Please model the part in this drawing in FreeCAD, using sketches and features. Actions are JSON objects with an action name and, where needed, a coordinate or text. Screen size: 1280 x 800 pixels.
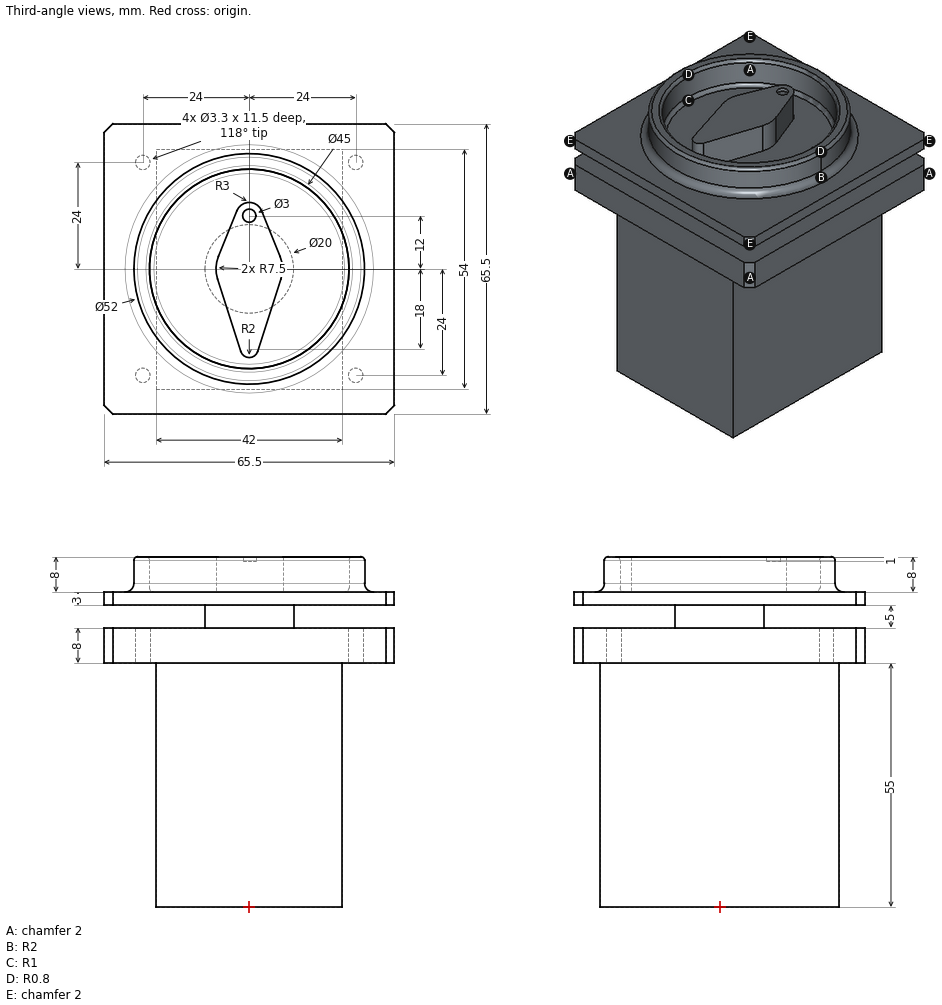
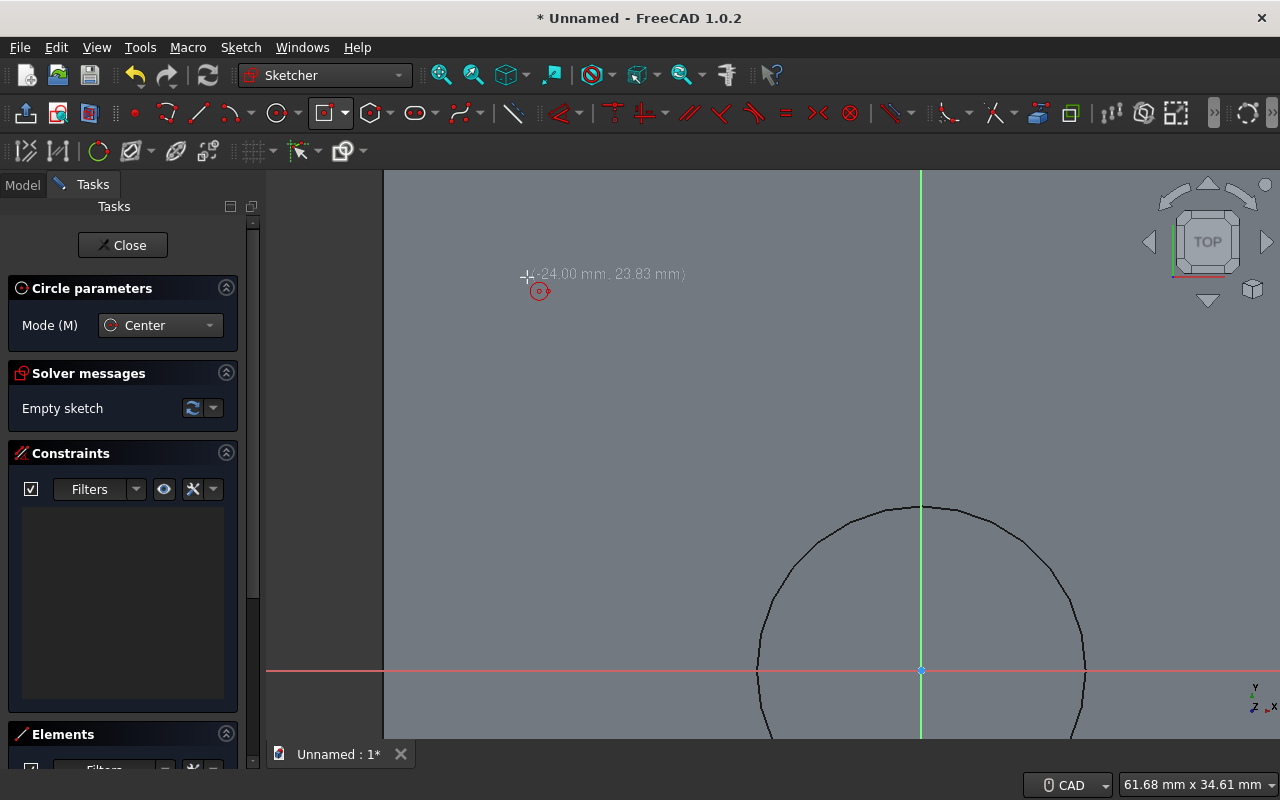
{"action": "left_click", "coordinate": [527, 276]}
{"action": "mouse_move", "coordinate": [546, 257]}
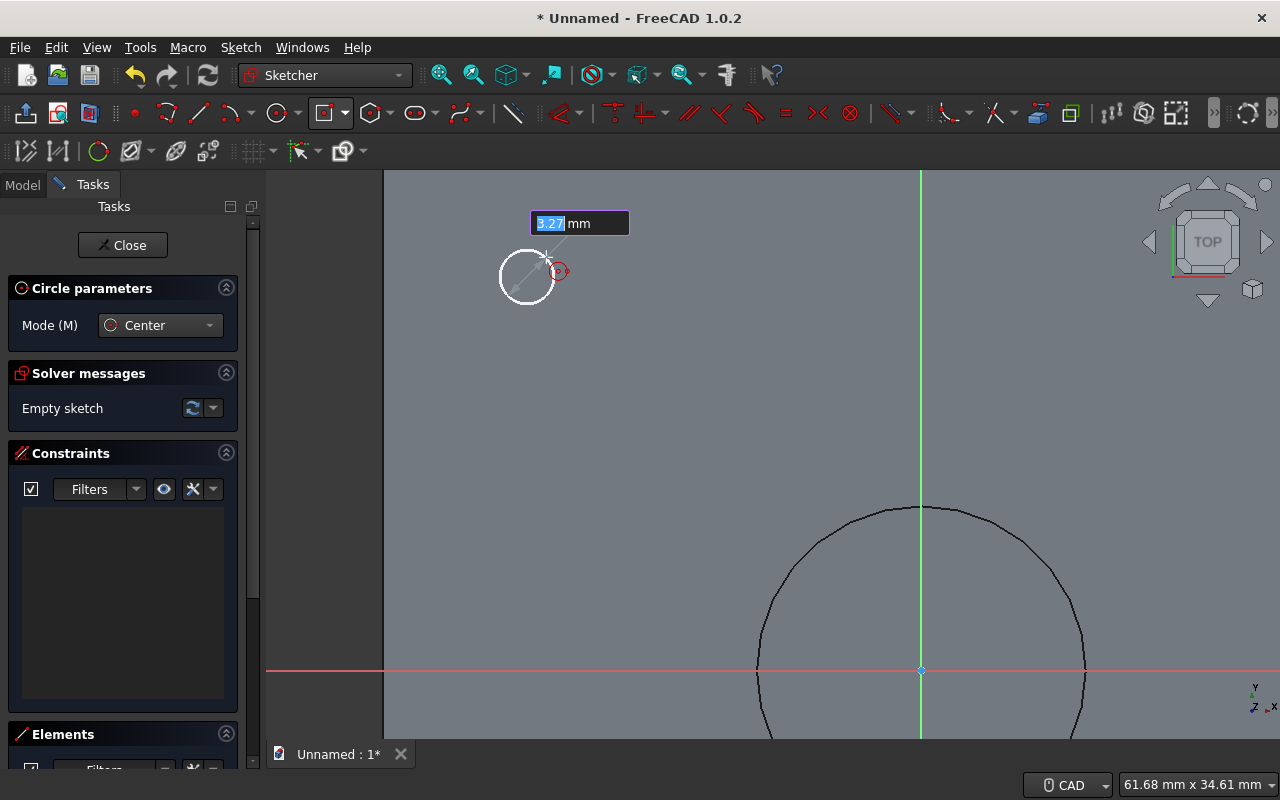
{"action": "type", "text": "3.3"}
{"action": "key", "text": "Return"}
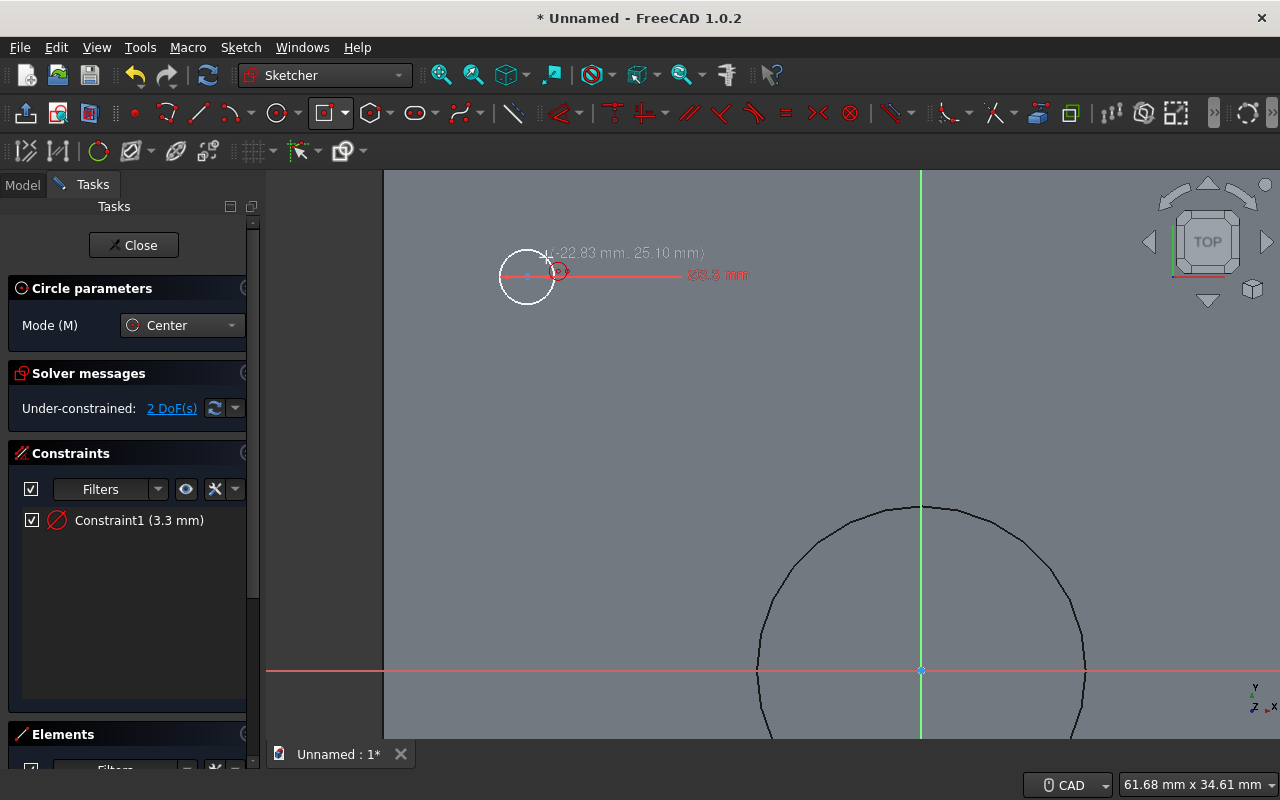
{"action": "scroll", "coordinate": [528, 278], "scroll_direction": "down", "scroll_amount": 4}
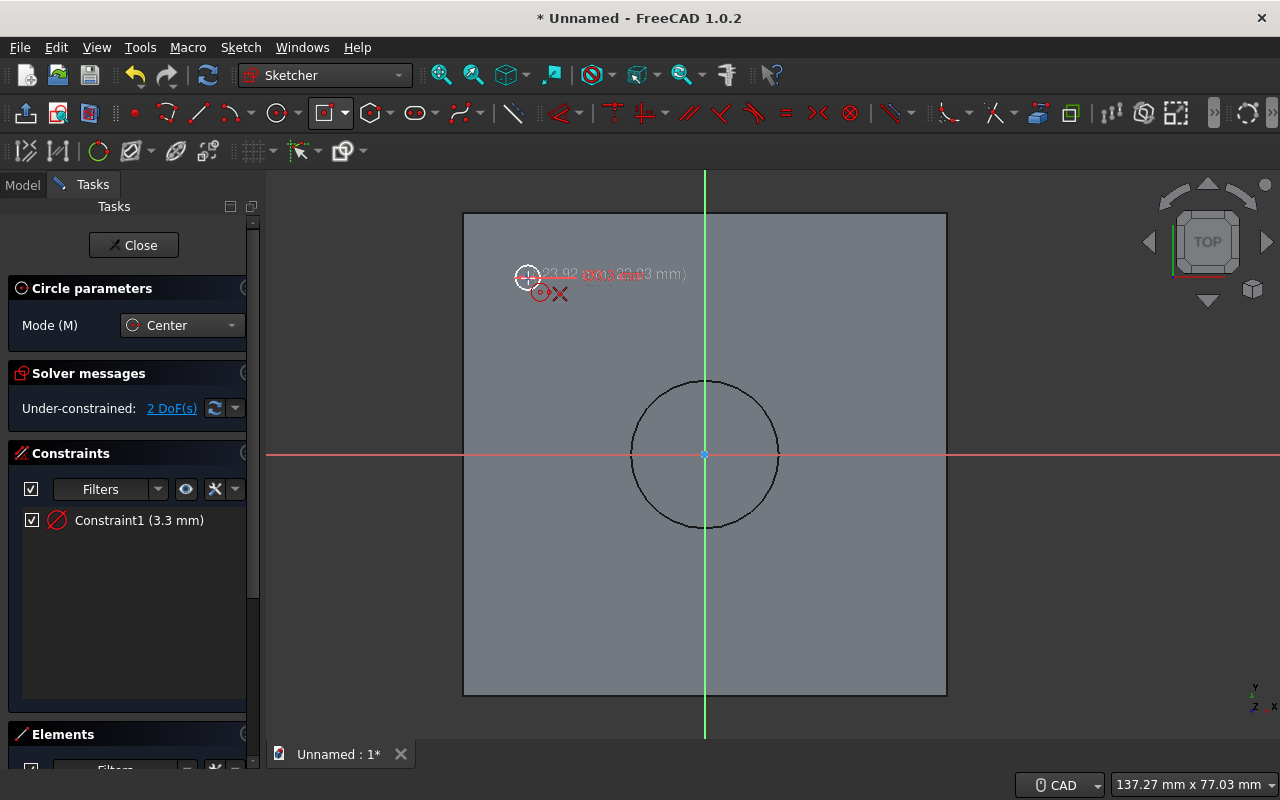
{"action": "scroll", "coordinate": [882, 277], "scroll_direction": "up", "scroll_amount": 4}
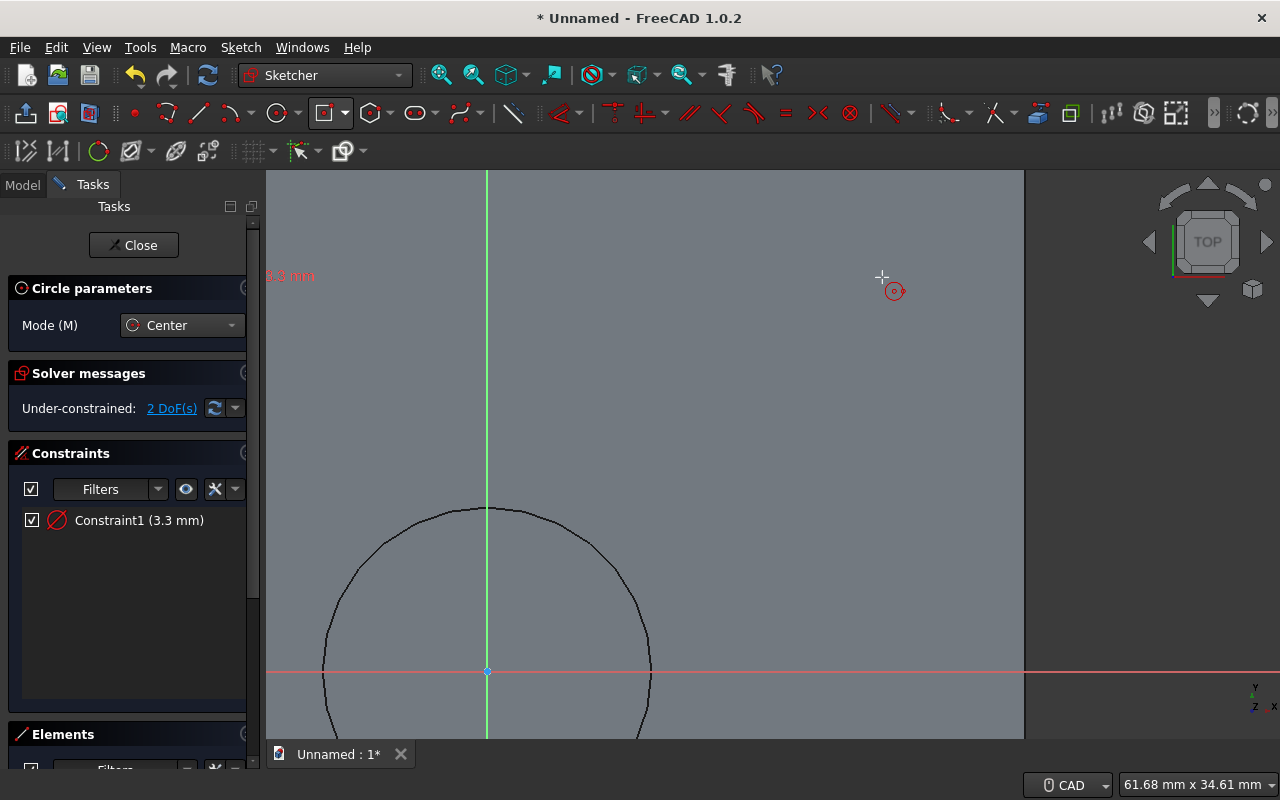
{"action": "left_click", "coordinate": [882, 277]}
{"action": "mouse_move", "coordinate": [901, 258]}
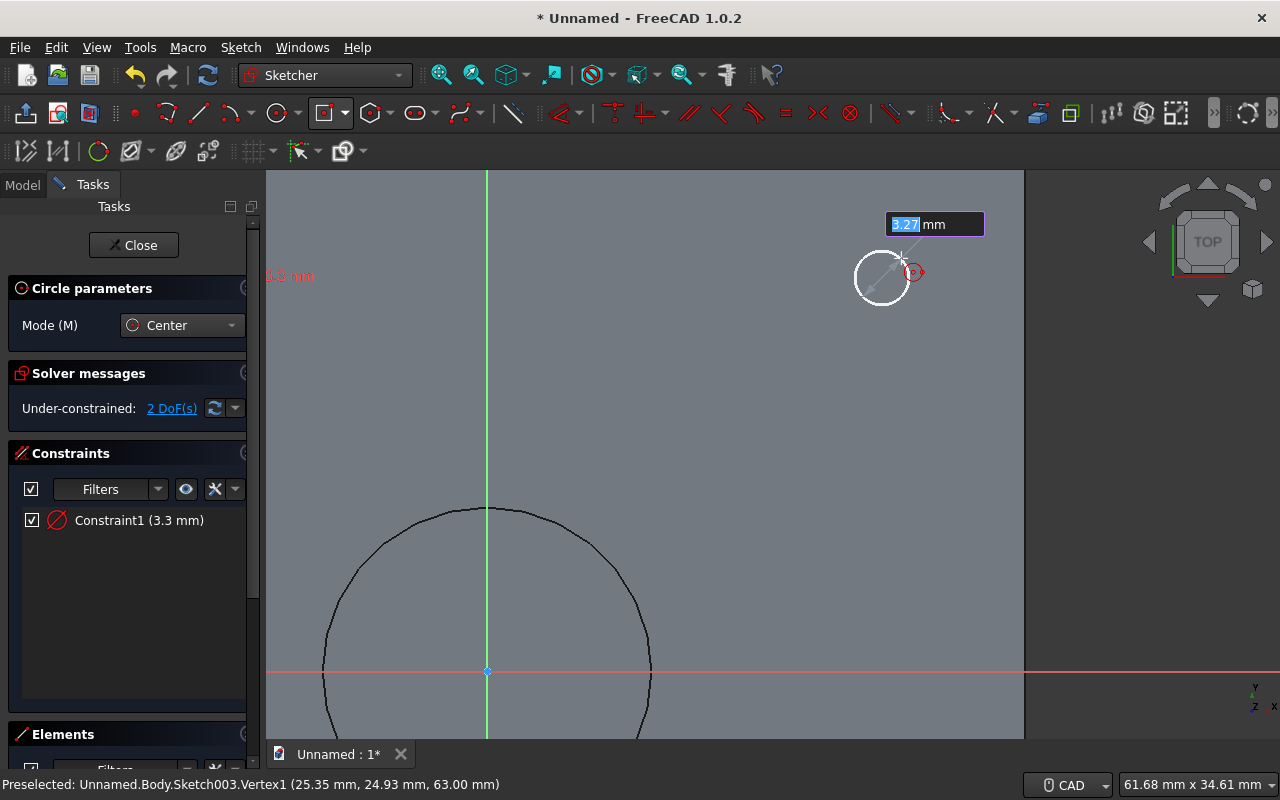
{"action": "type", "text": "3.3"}
{"action": "key", "text": "Return"}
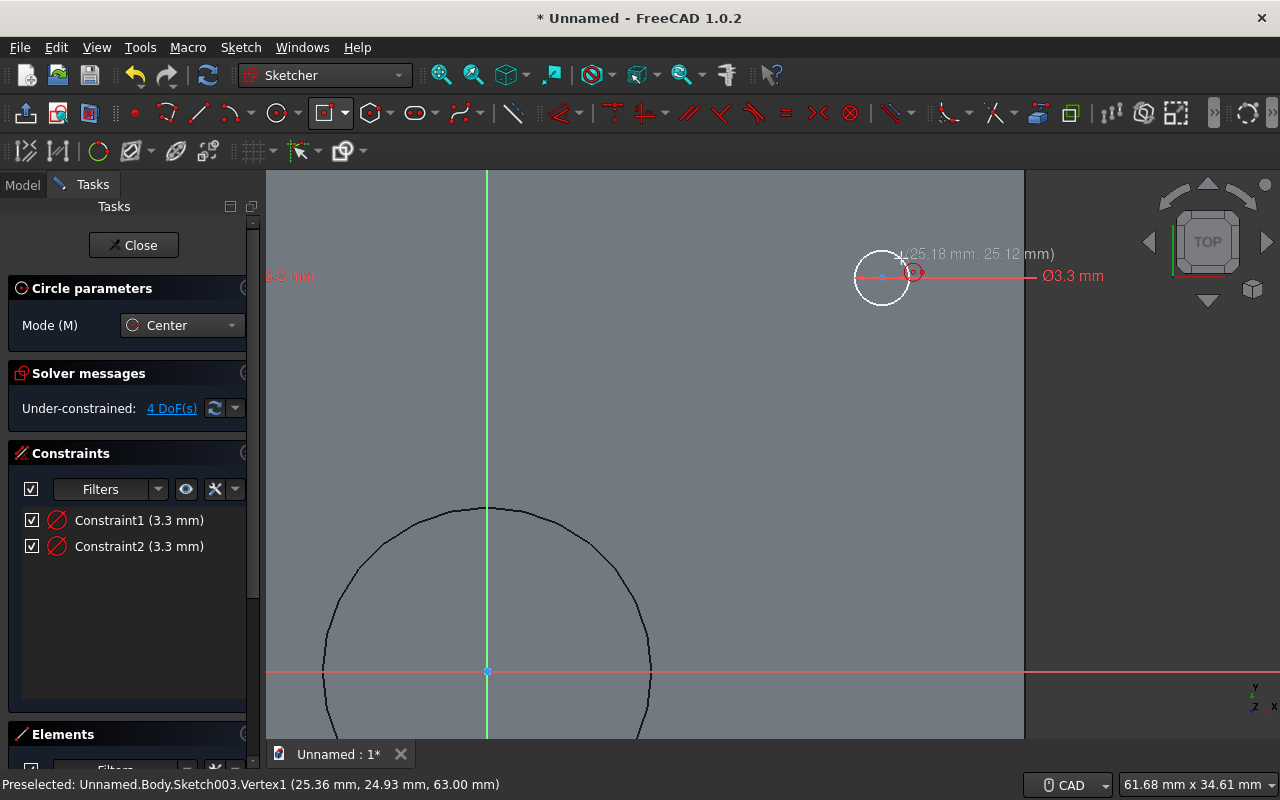
{"action": "scroll", "coordinate": [882, 277], "scroll_direction": "down", "scroll_amount": 4}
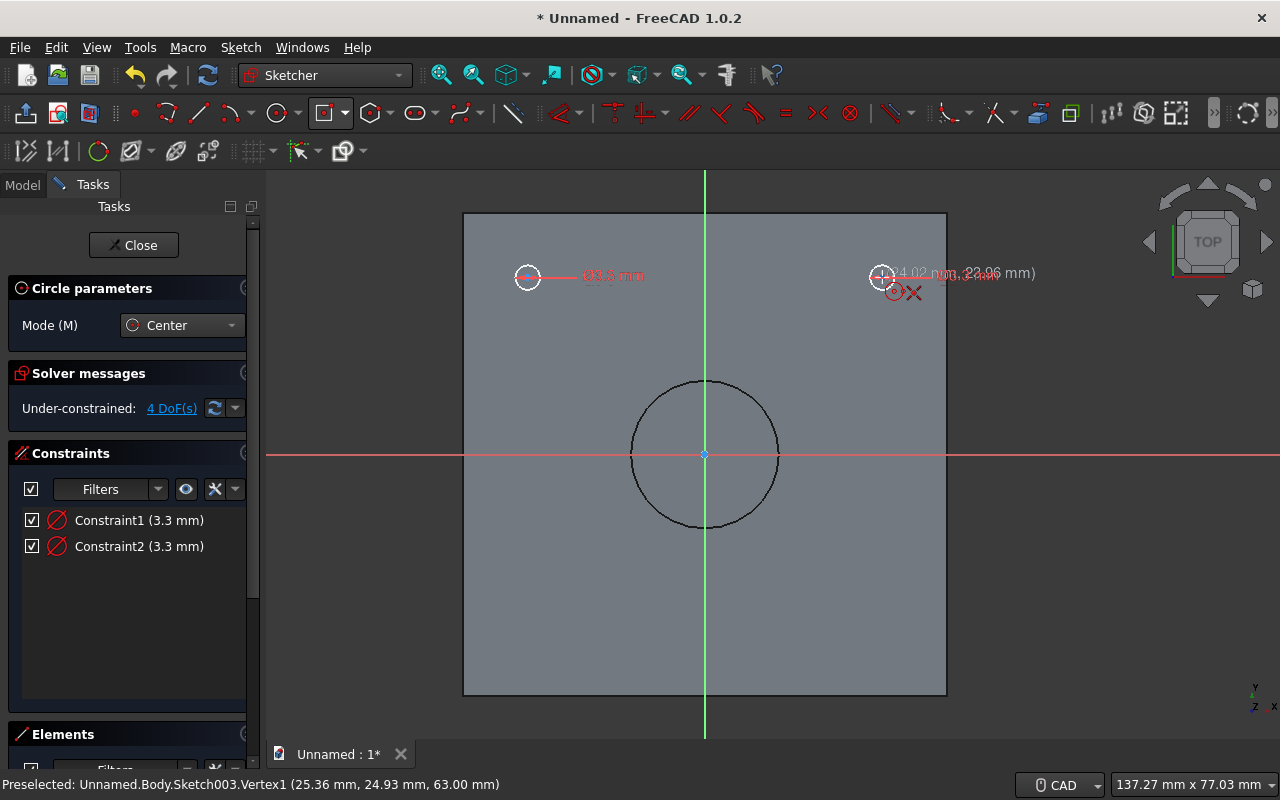
{"action": "scroll", "coordinate": [882, 632], "scroll_direction": "up", "scroll_amount": 4}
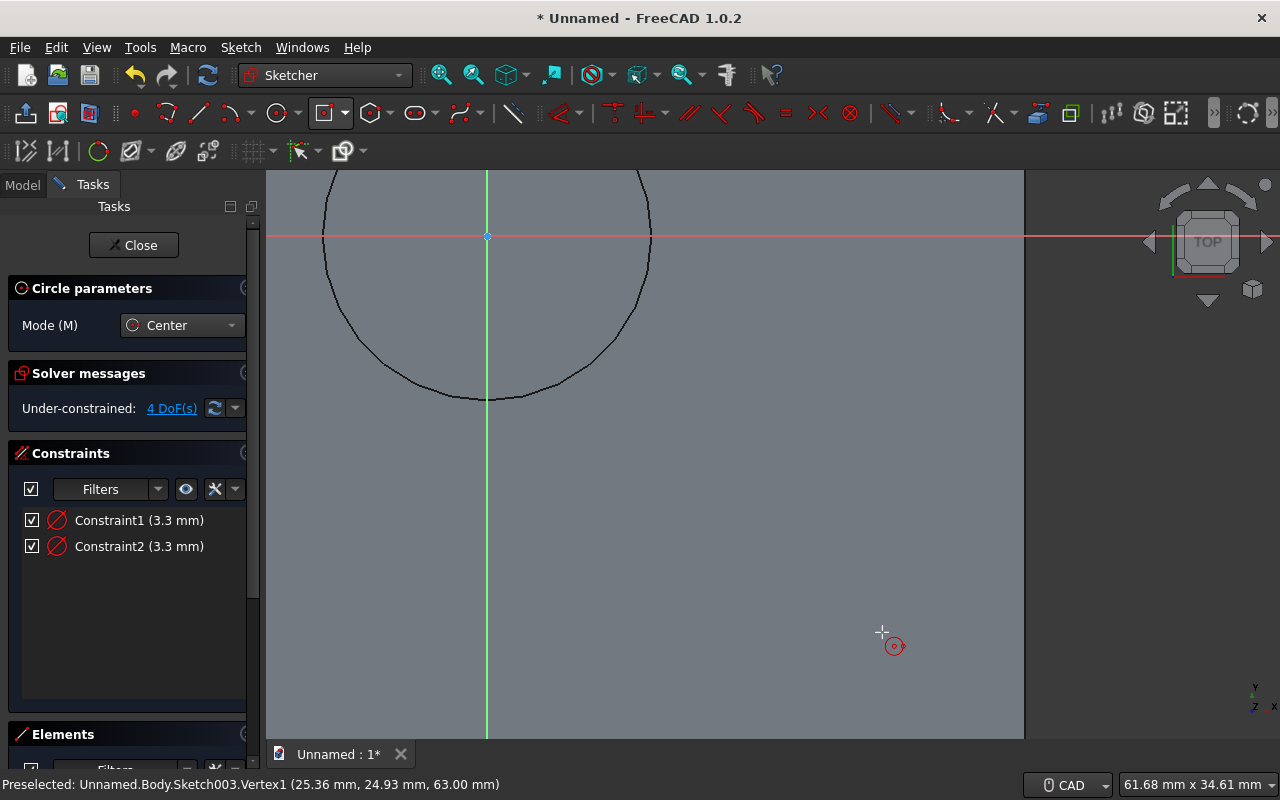
{"action": "left_click", "coordinate": [882, 631]}
{"action": "mouse_move", "coordinate": [901, 611]}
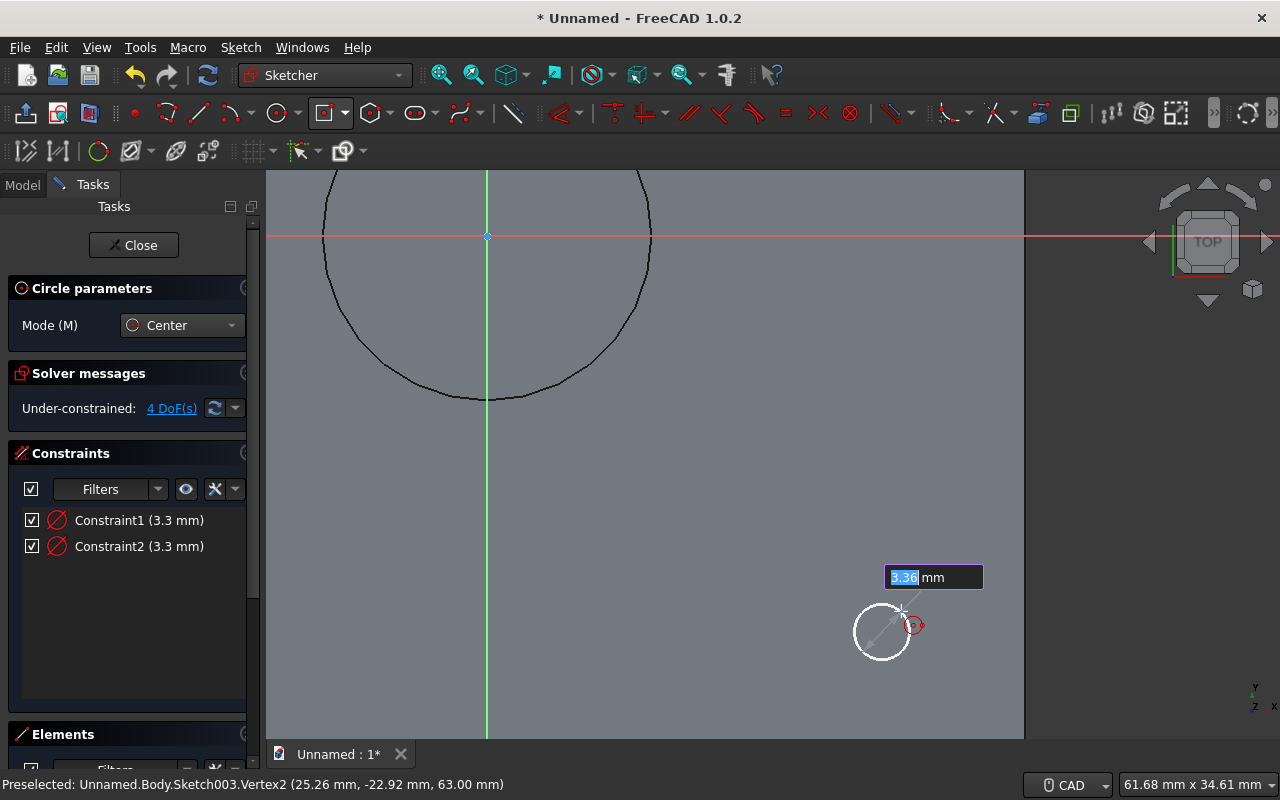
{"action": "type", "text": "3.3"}
{"action": "key", "text": "Return"}